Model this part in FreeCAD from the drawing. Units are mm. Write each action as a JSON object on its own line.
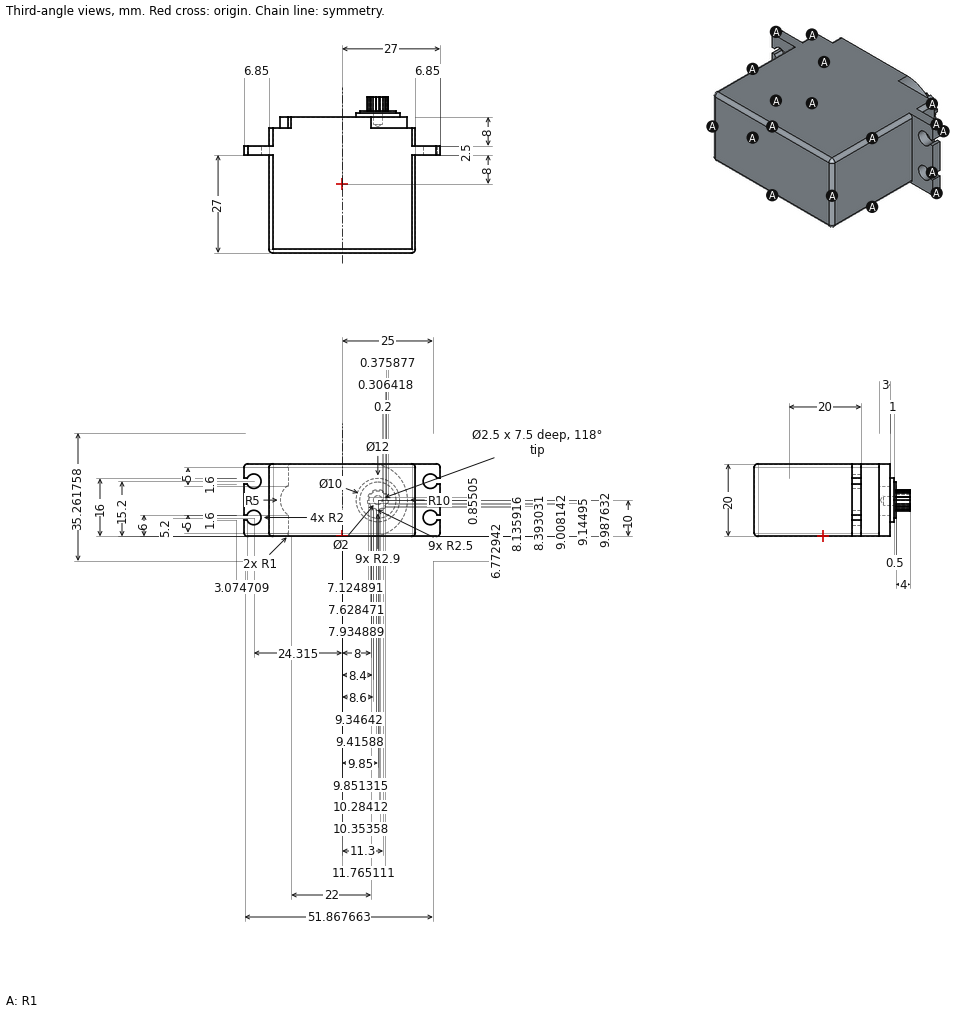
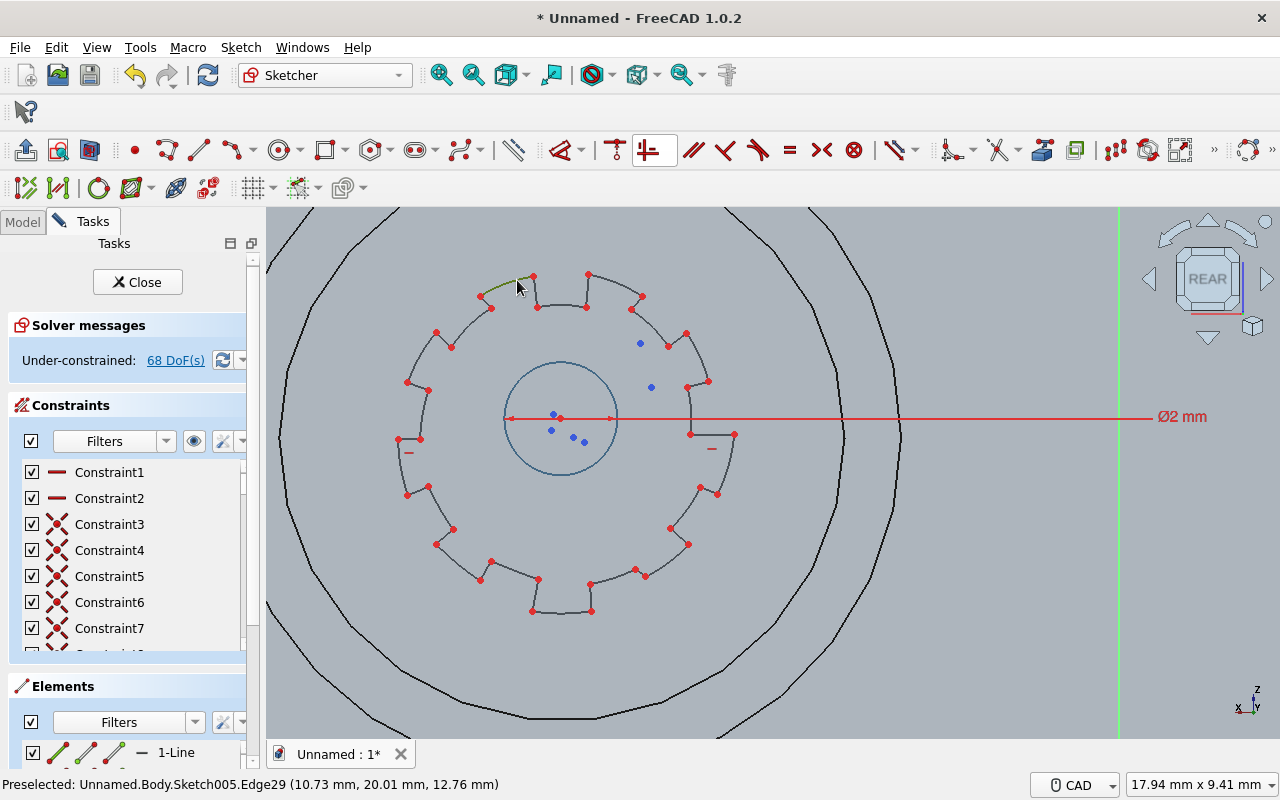
{"action": "left_click", "coordinate": [616, 150]}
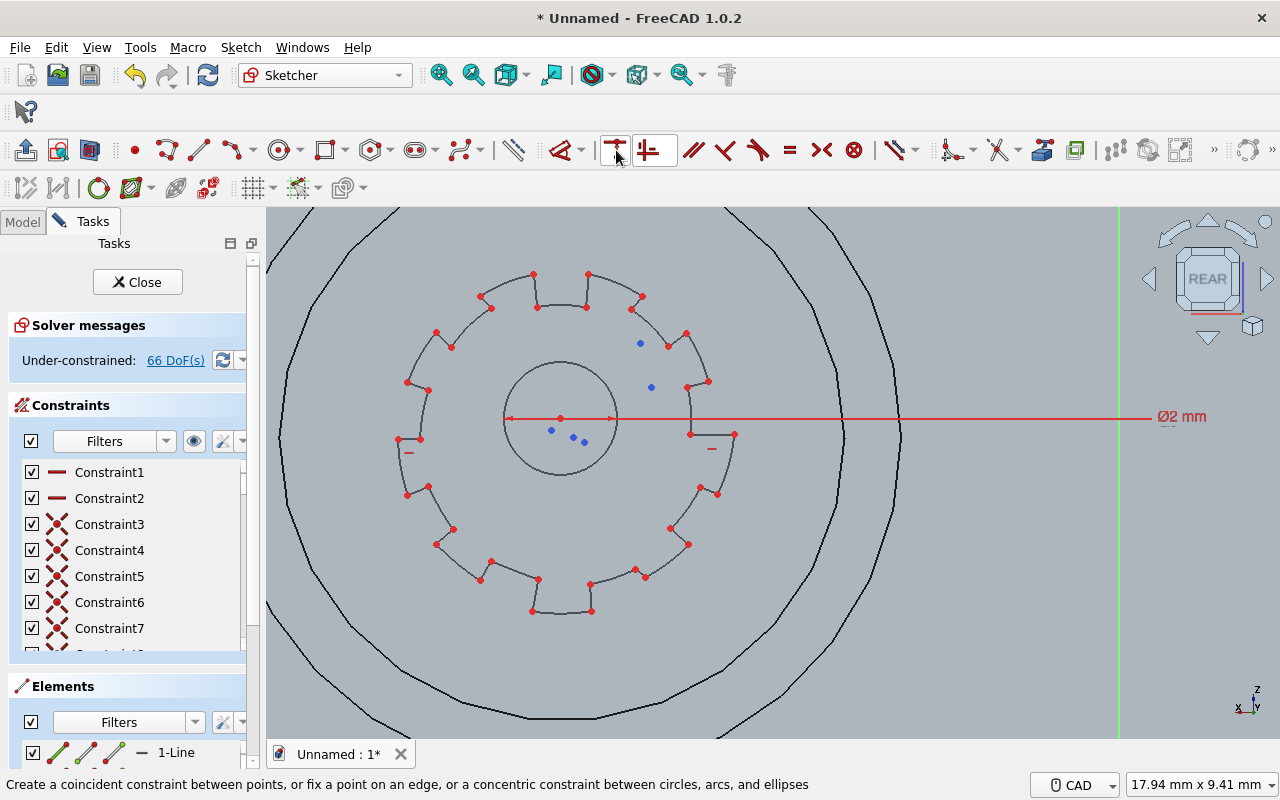
{"action": "left_click", "coordinate": [600, 378]}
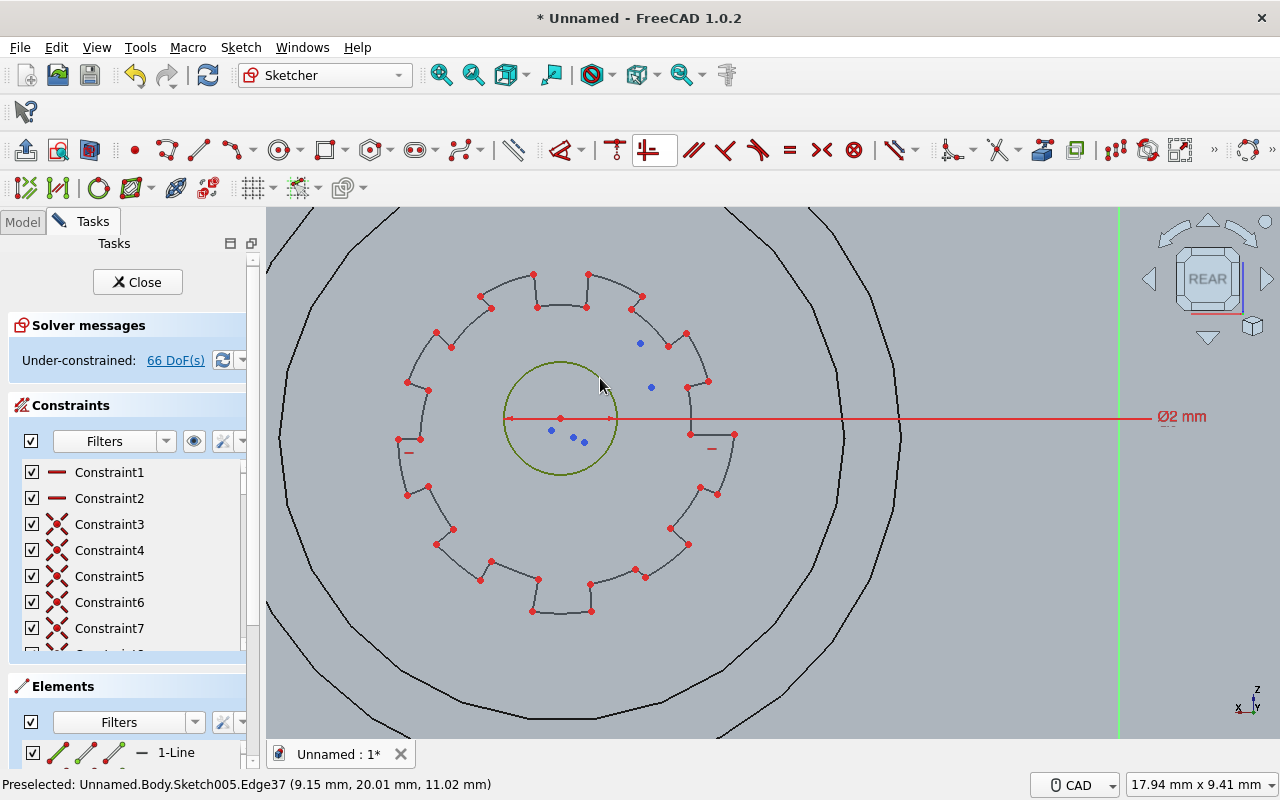
{"action": "left_click", "coordinate": [426, 347]}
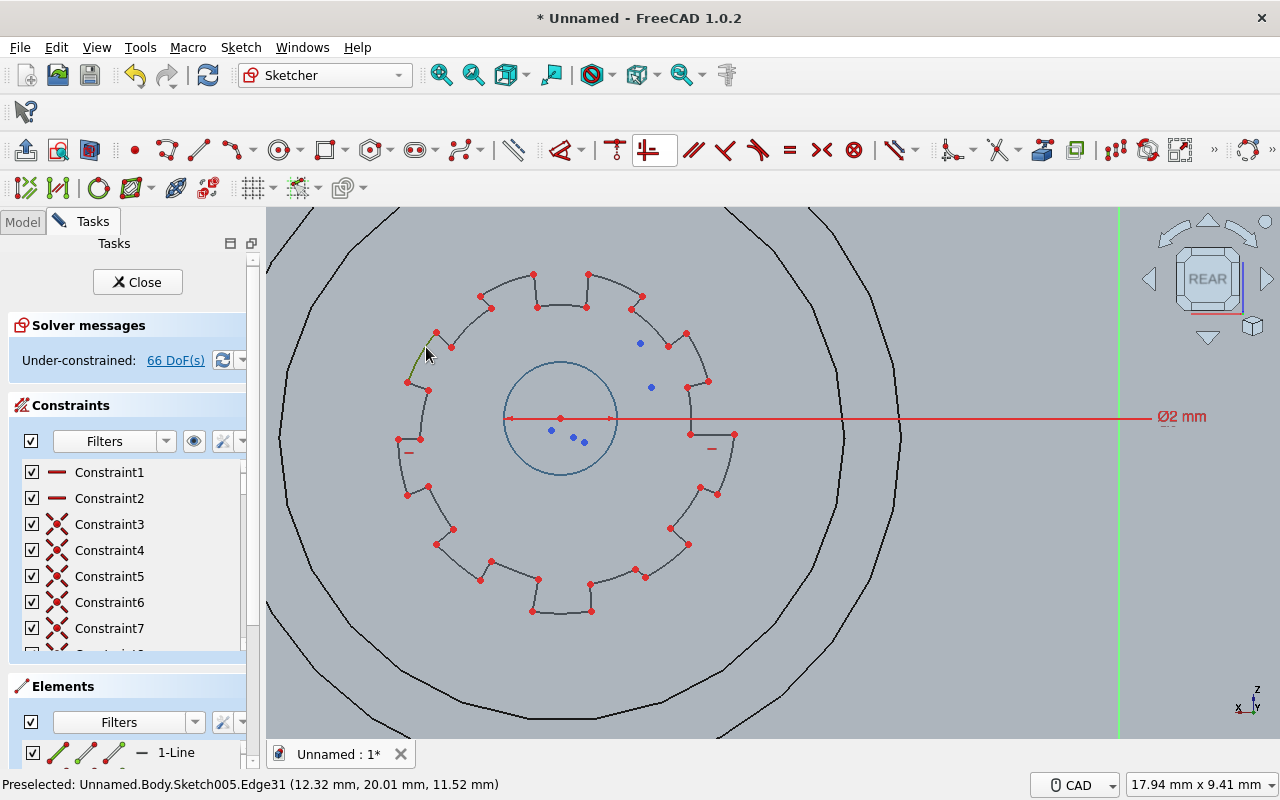
{"action": "left_click", "coordinate": [616, 150]}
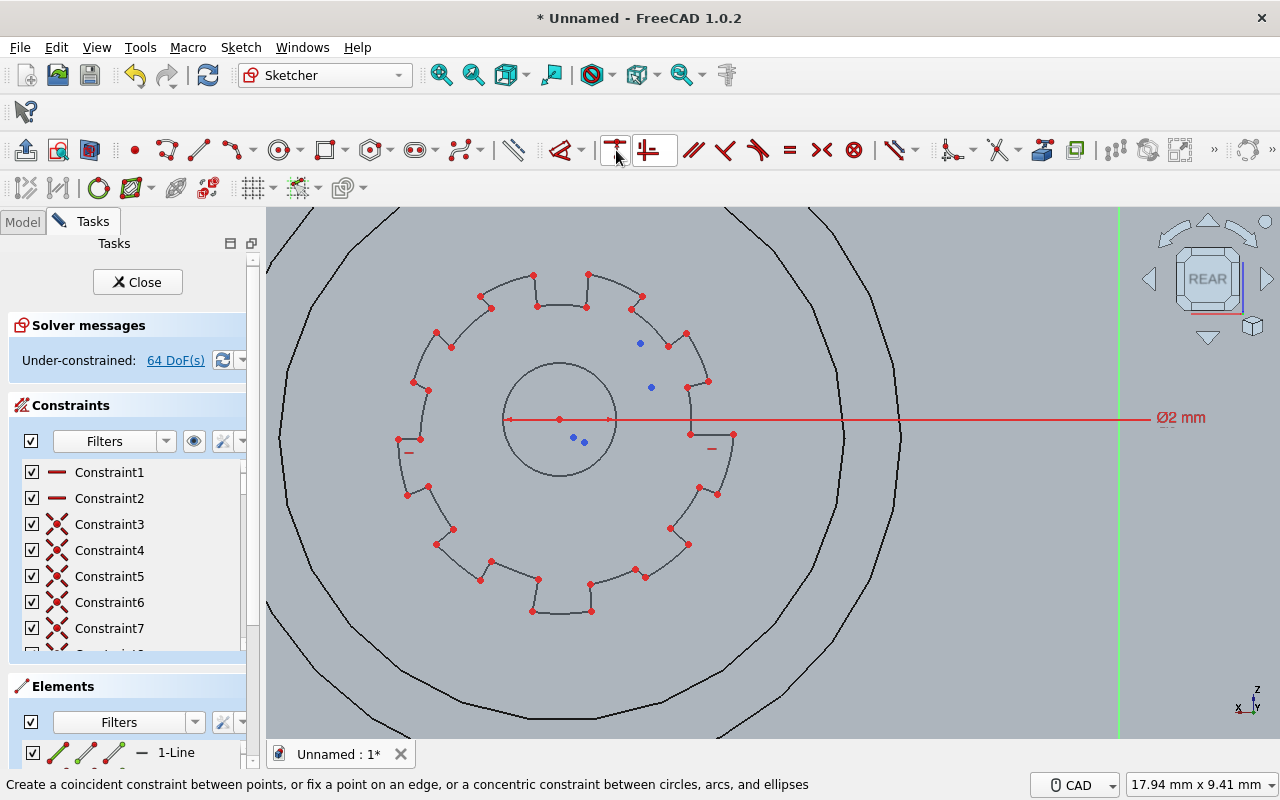
{"action": "left_click", "coordinate": [599, 379]}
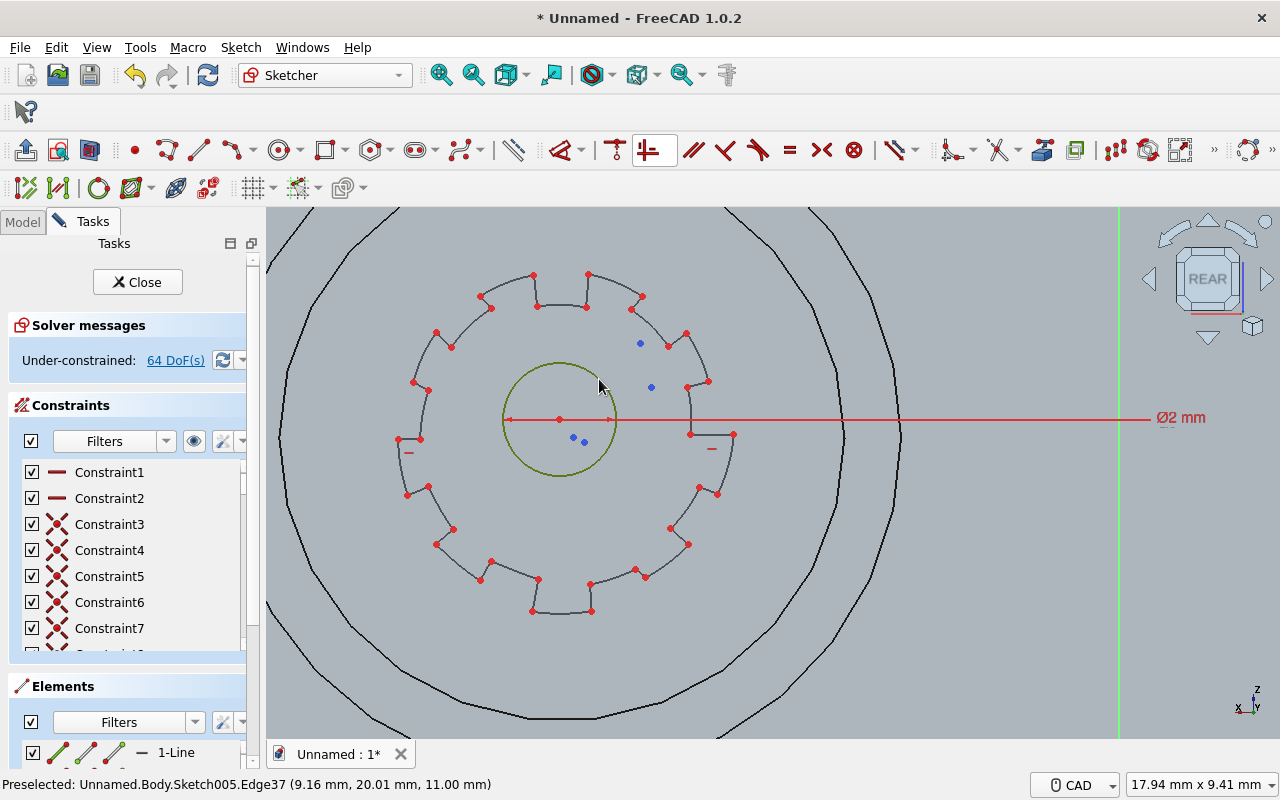
{"action": "left_click", "coordinate": [425, 405]}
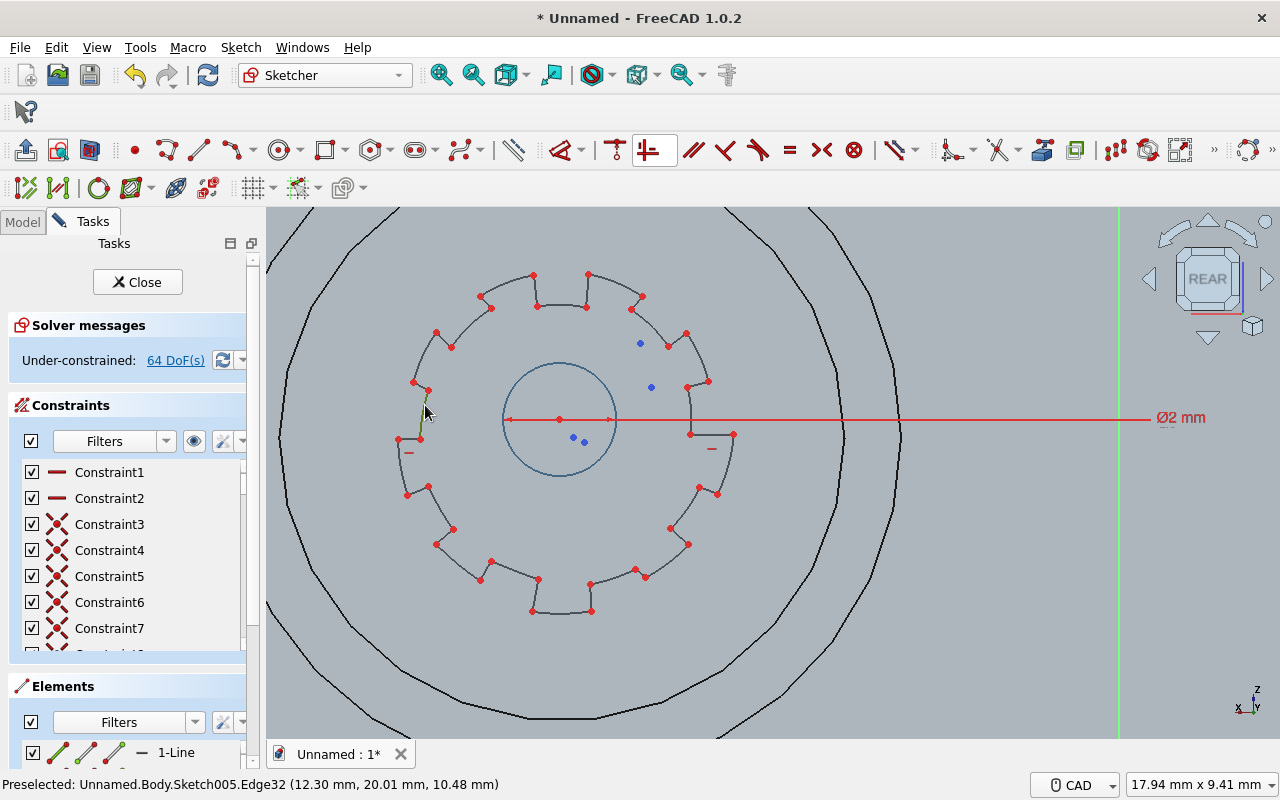
{"action": "left_click", "coordinate": [616, 150]}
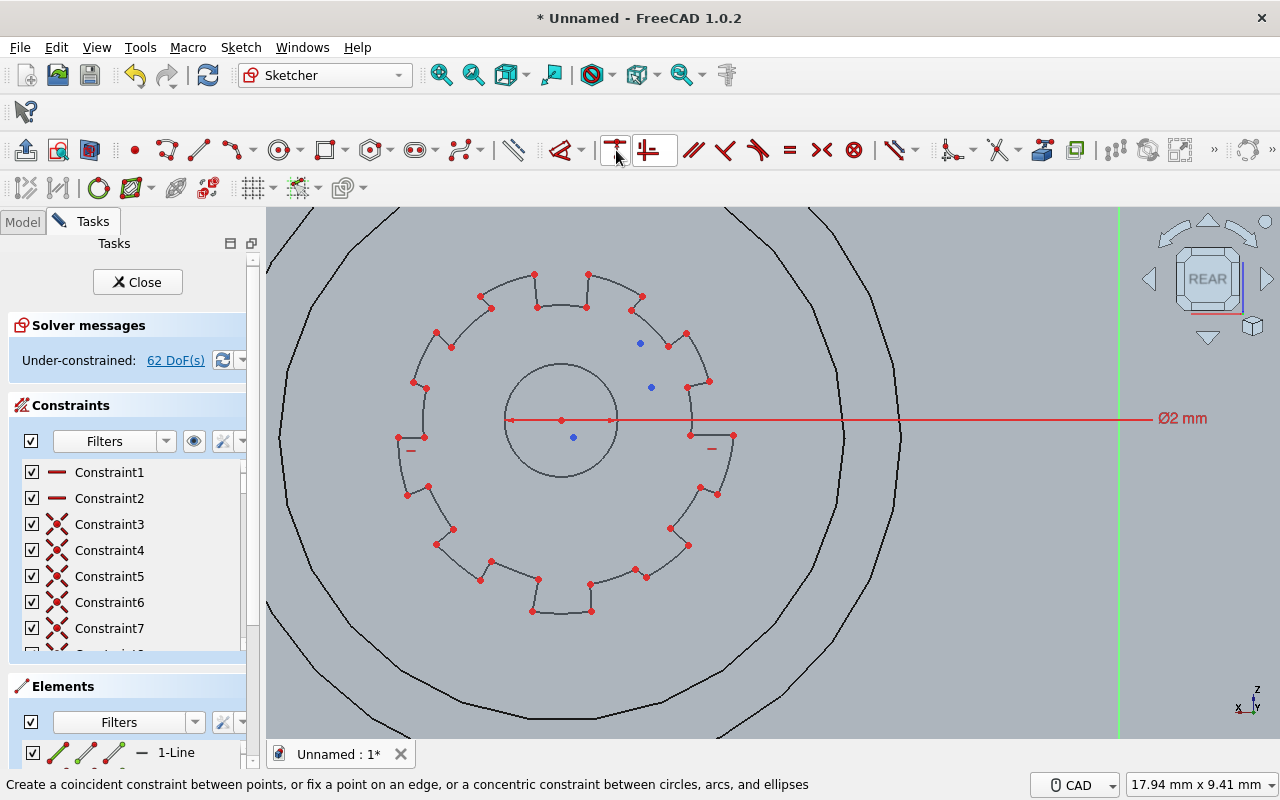
{"action": "left_click", "coordinate": [601, 380]}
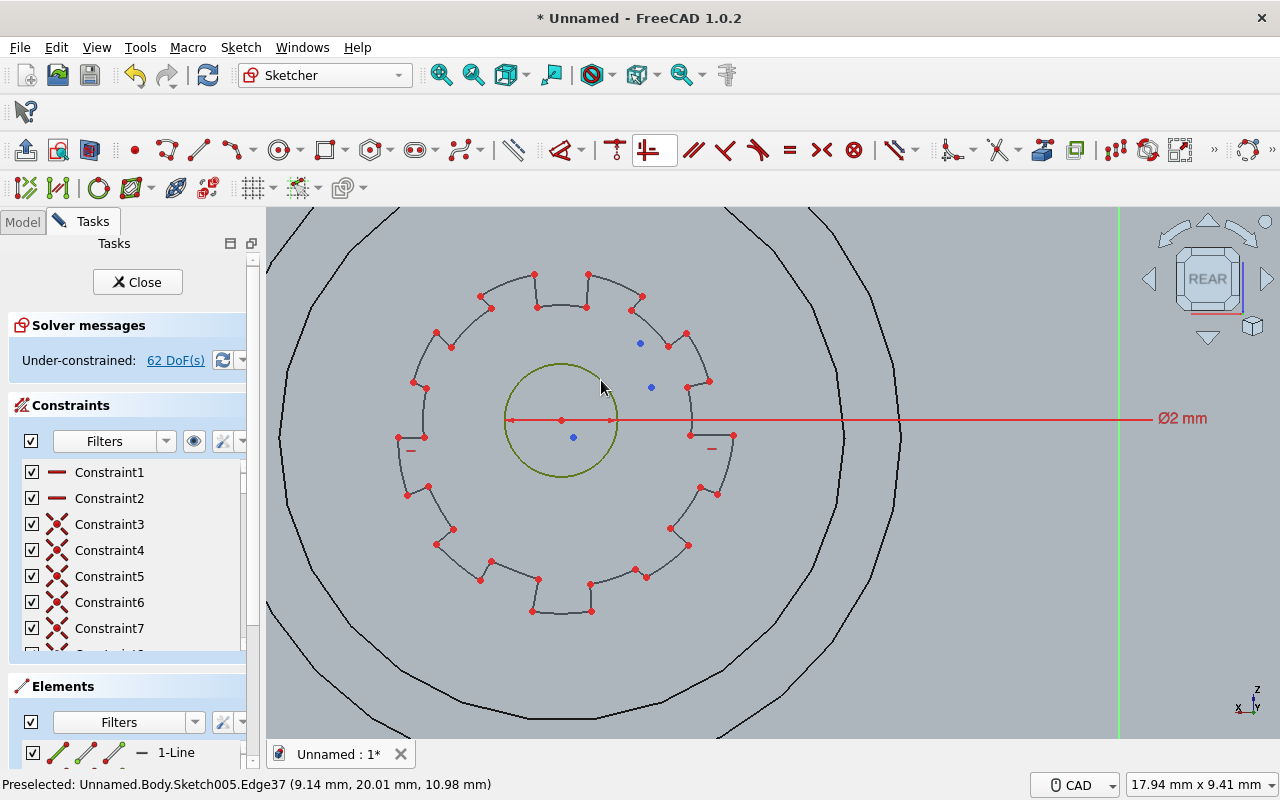
{"action": "left_click", "coordinate": [399, 455]}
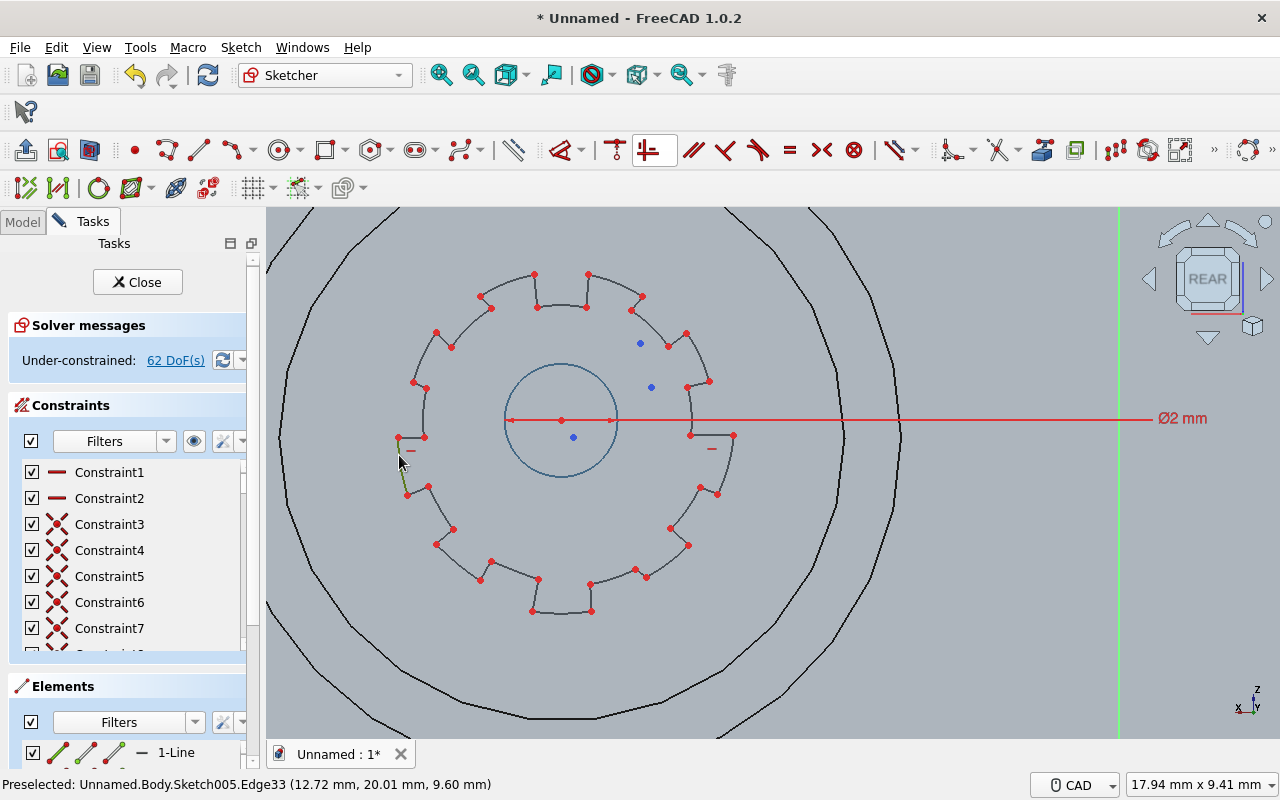
{"action": "left_click", "coordinate": [616, 150]}